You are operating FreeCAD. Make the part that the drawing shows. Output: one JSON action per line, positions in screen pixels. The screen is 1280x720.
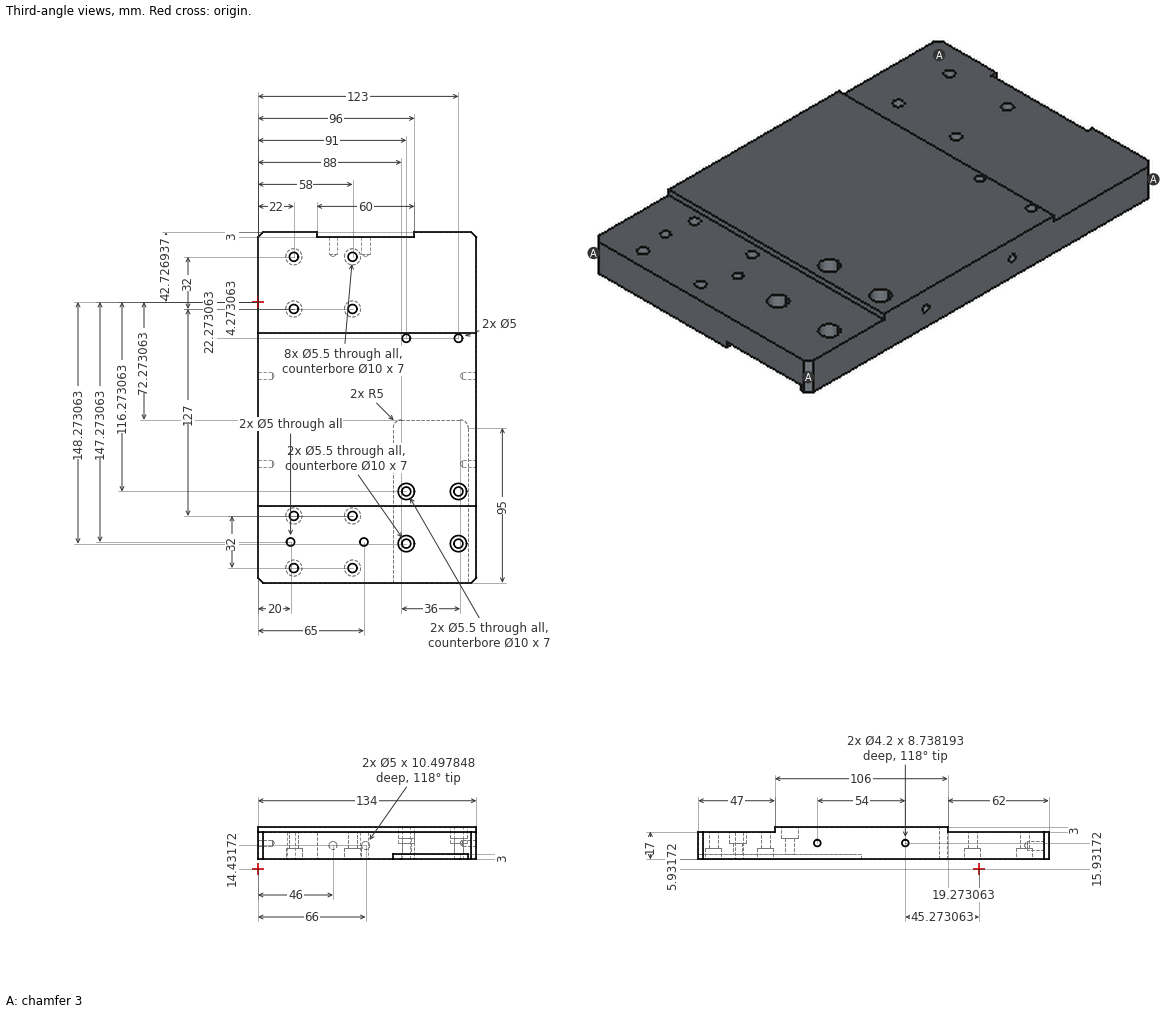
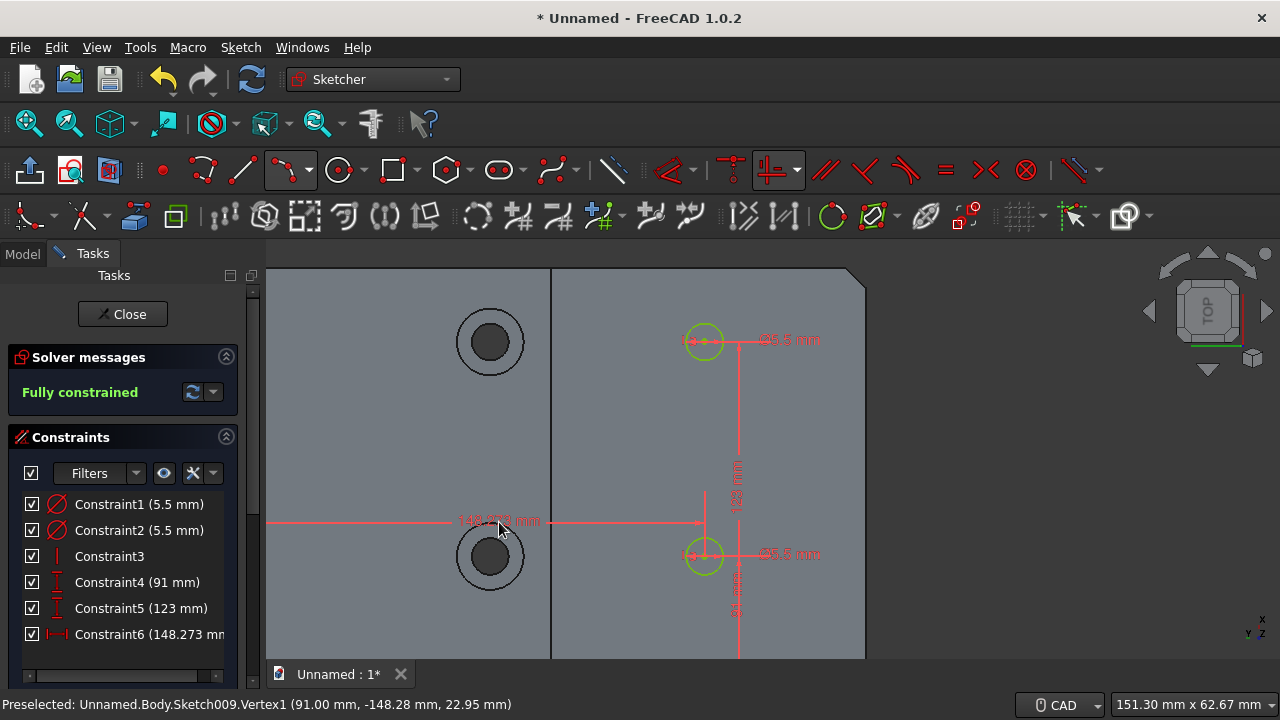
{"action": "left_click", "coordinate": [123, 314]}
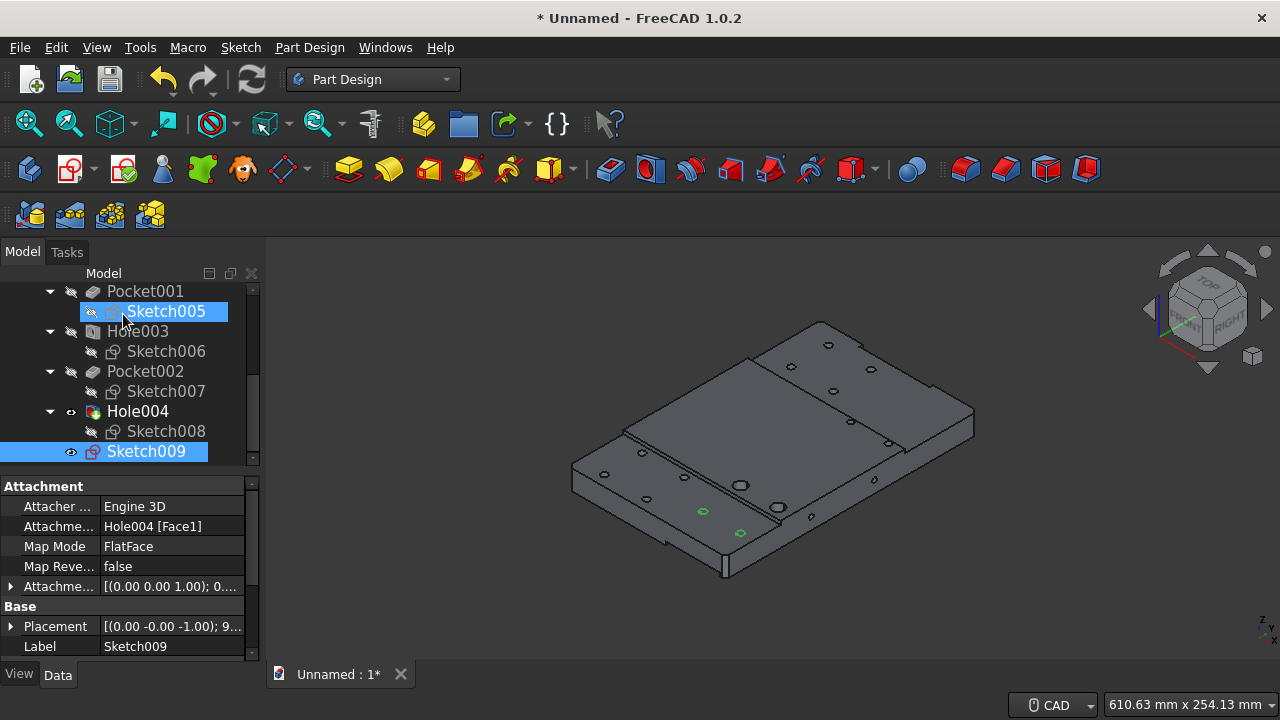
{"action": "left_click", "coordinate": [652, 170]}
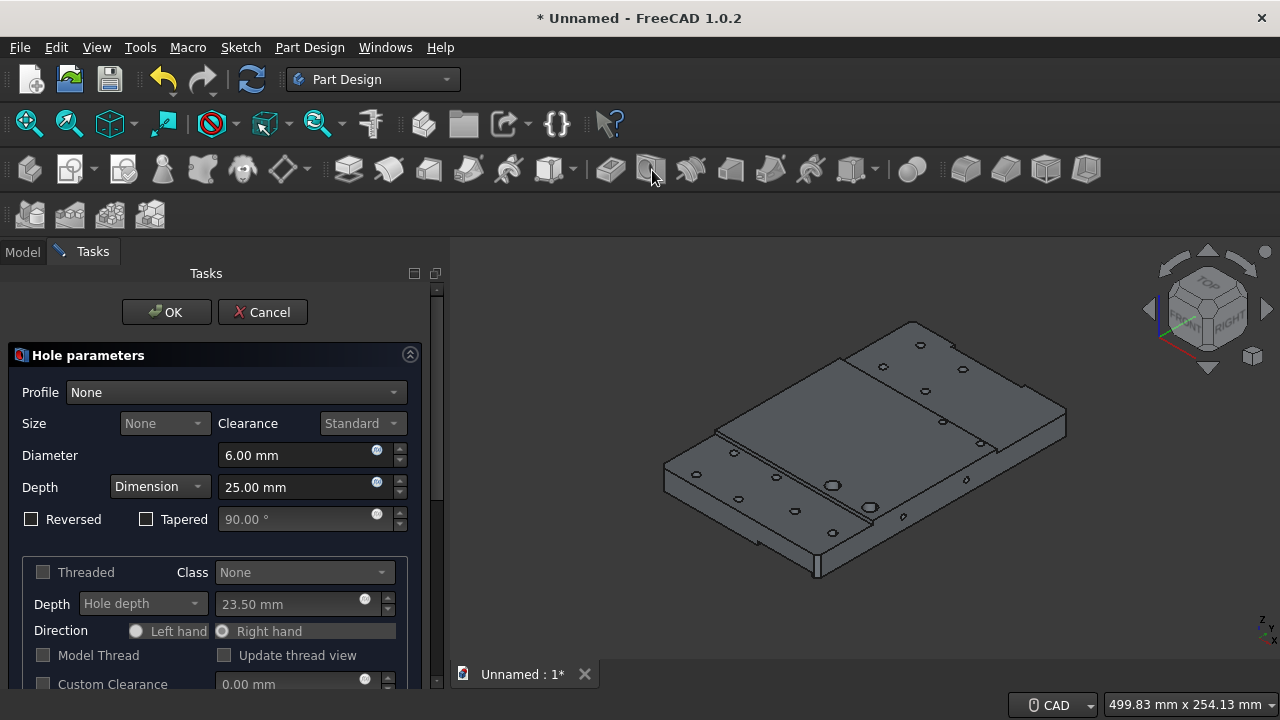
{"action": "triple_click", "coordinate": [305, 455]}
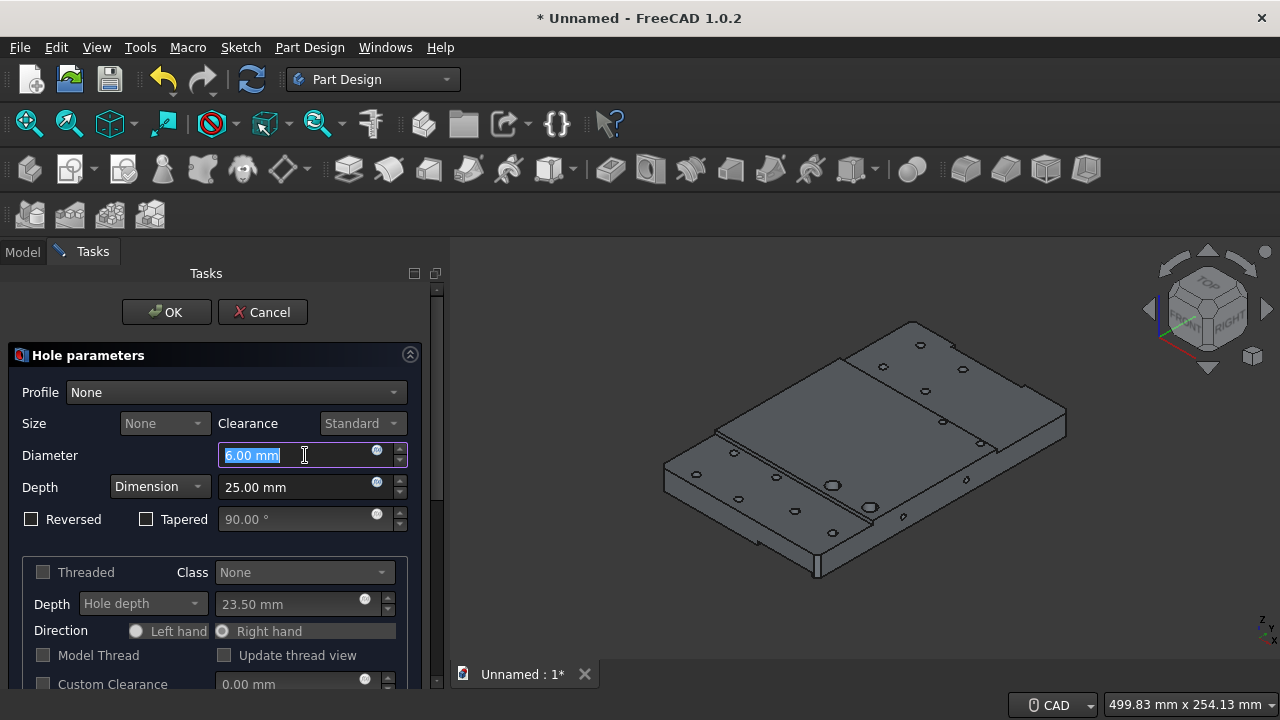
{"action": "type", "text": "5.5"}
{"action": "key", "text": "Tab"}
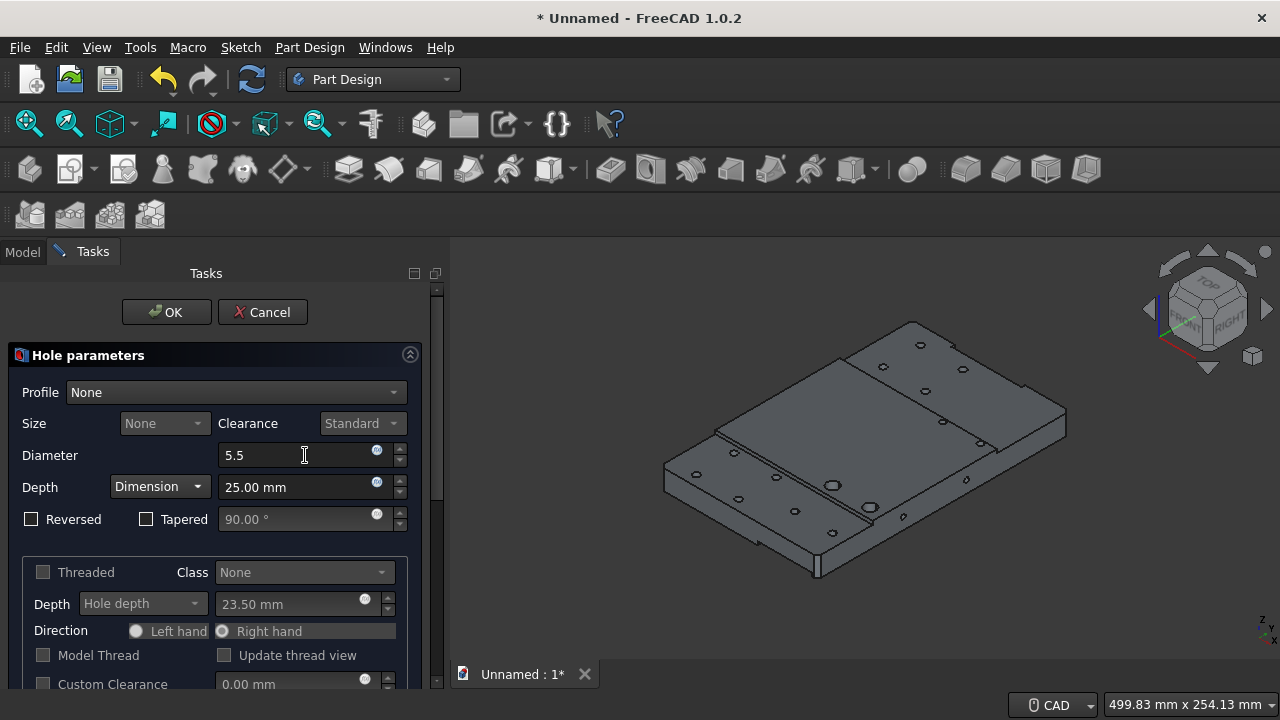
{"action": "left_click", "coordinate": [161, 486]}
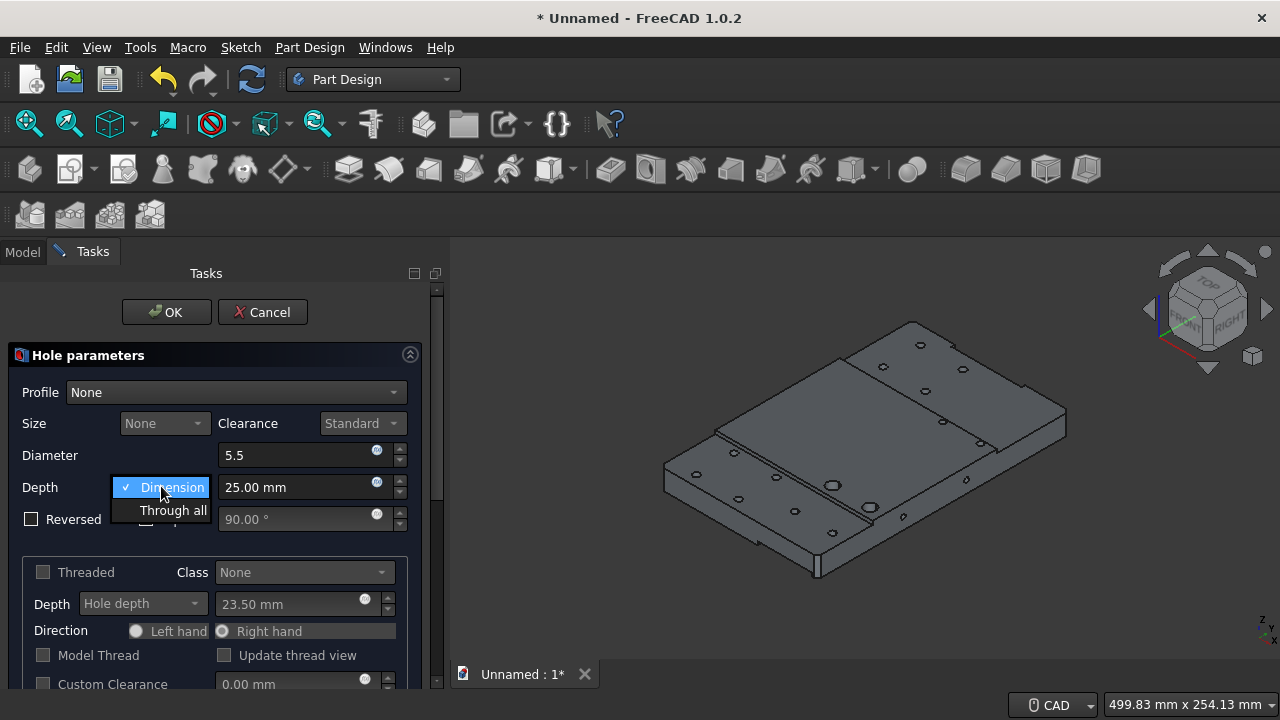
{"action": "left_click", "coordinate": [160, 510]}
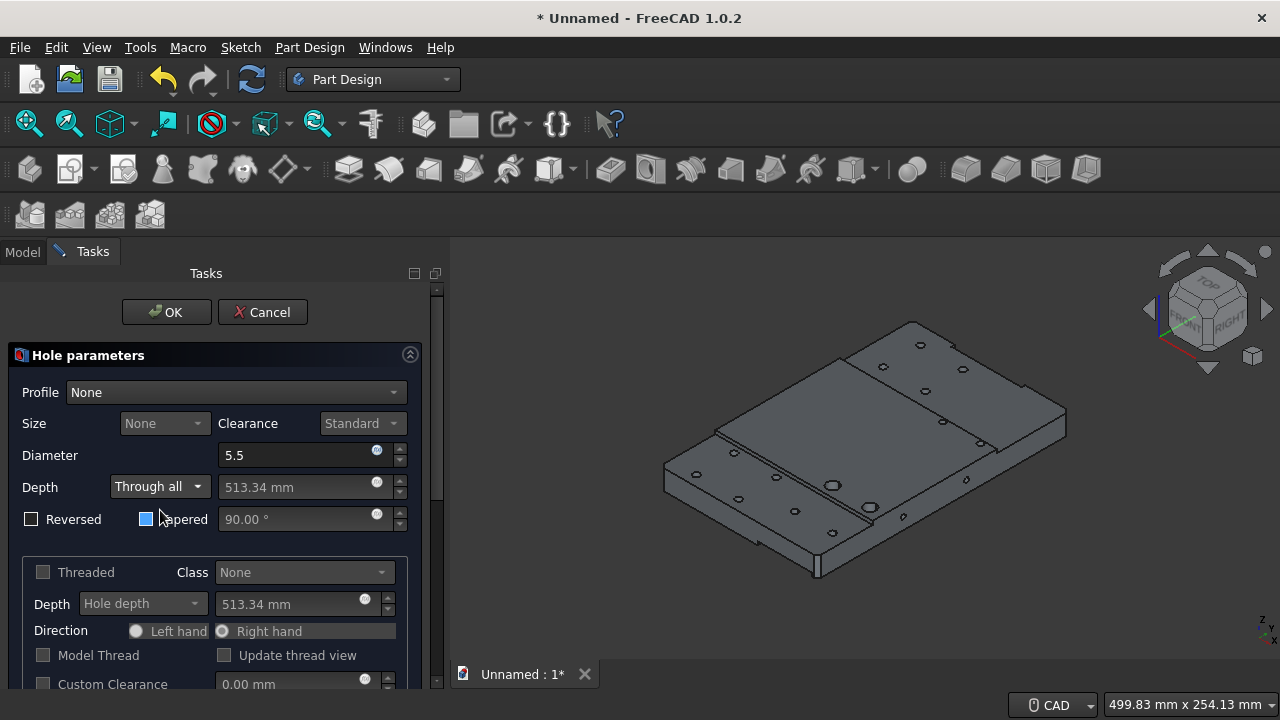
{"action": "scroll", "coordinate": [437, 486], "scroll_direction": "down", "scroll_amount": 3}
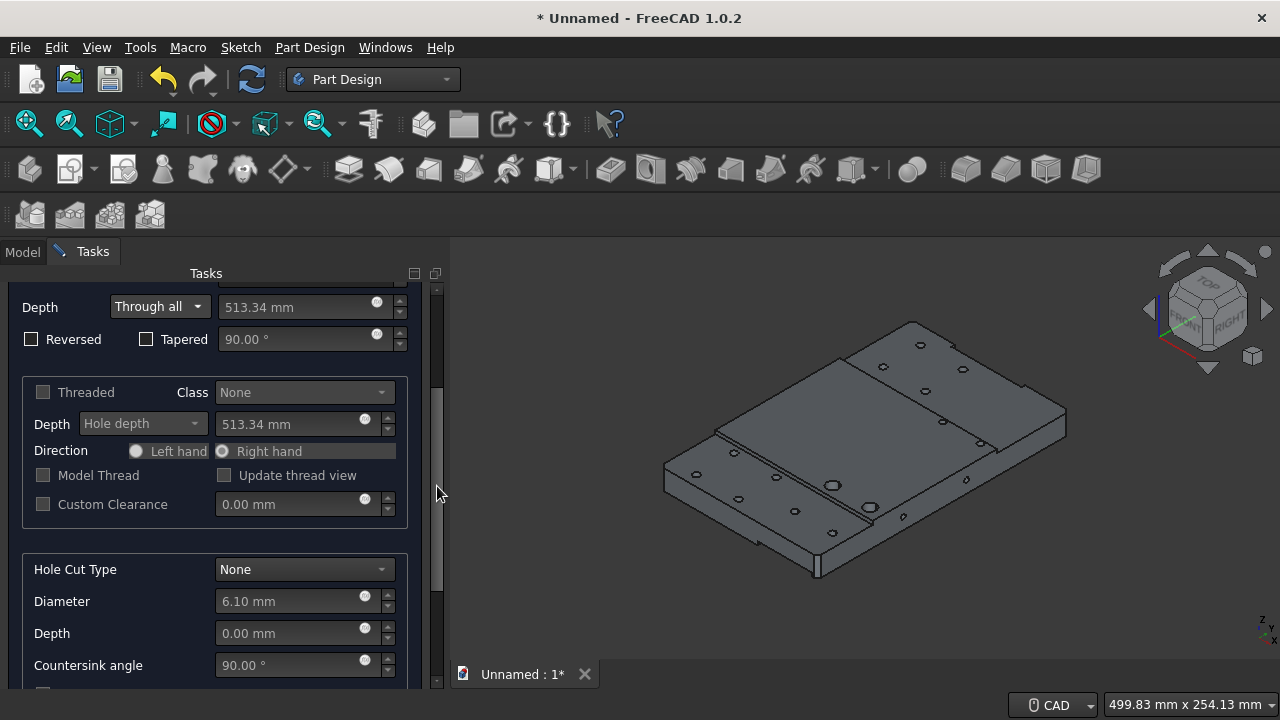
{"action": "left_click", "coordinate": [306, 570]}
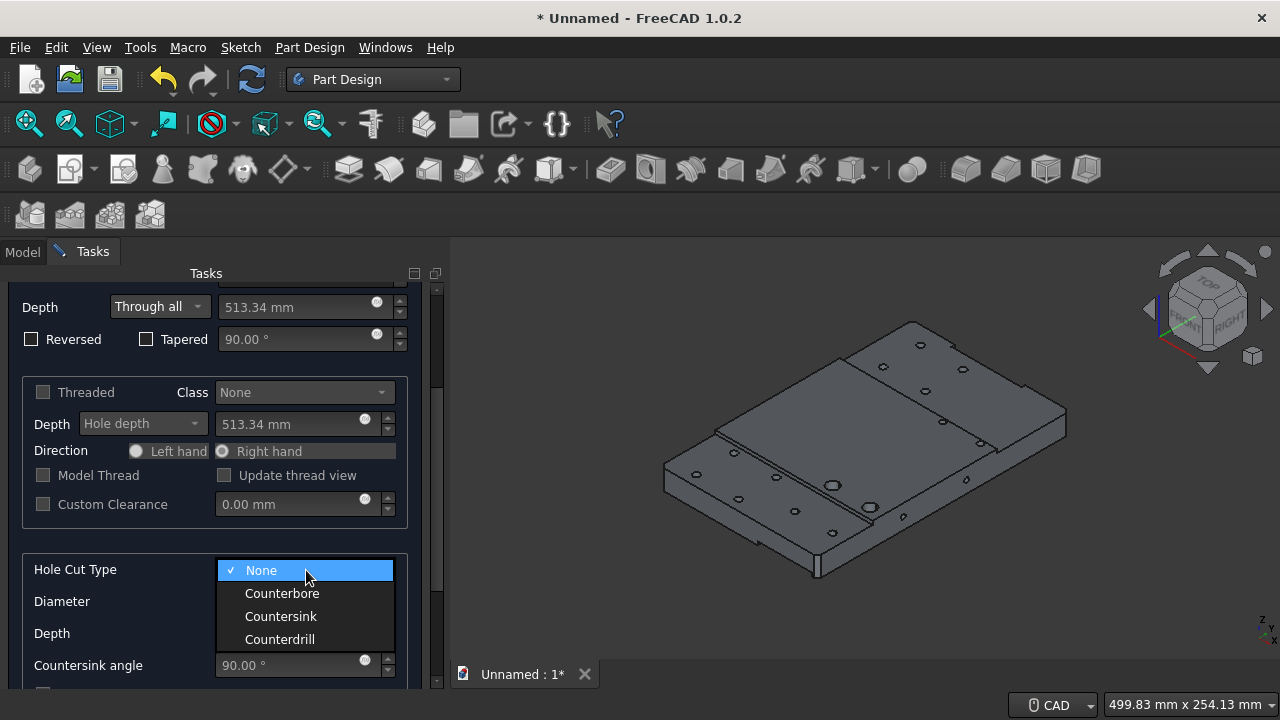
{"action": "left_click", "coordinate": [304, 594]}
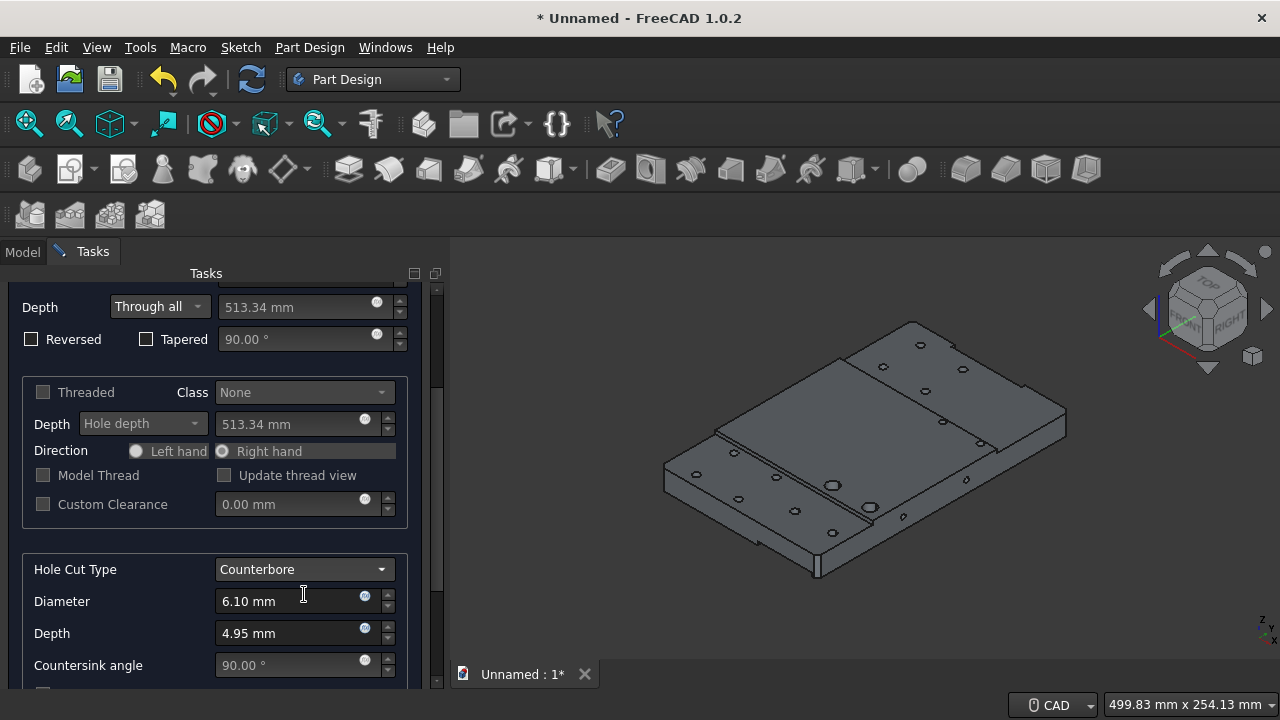
{"action": "triple_click", "coordinate": [298, 601]}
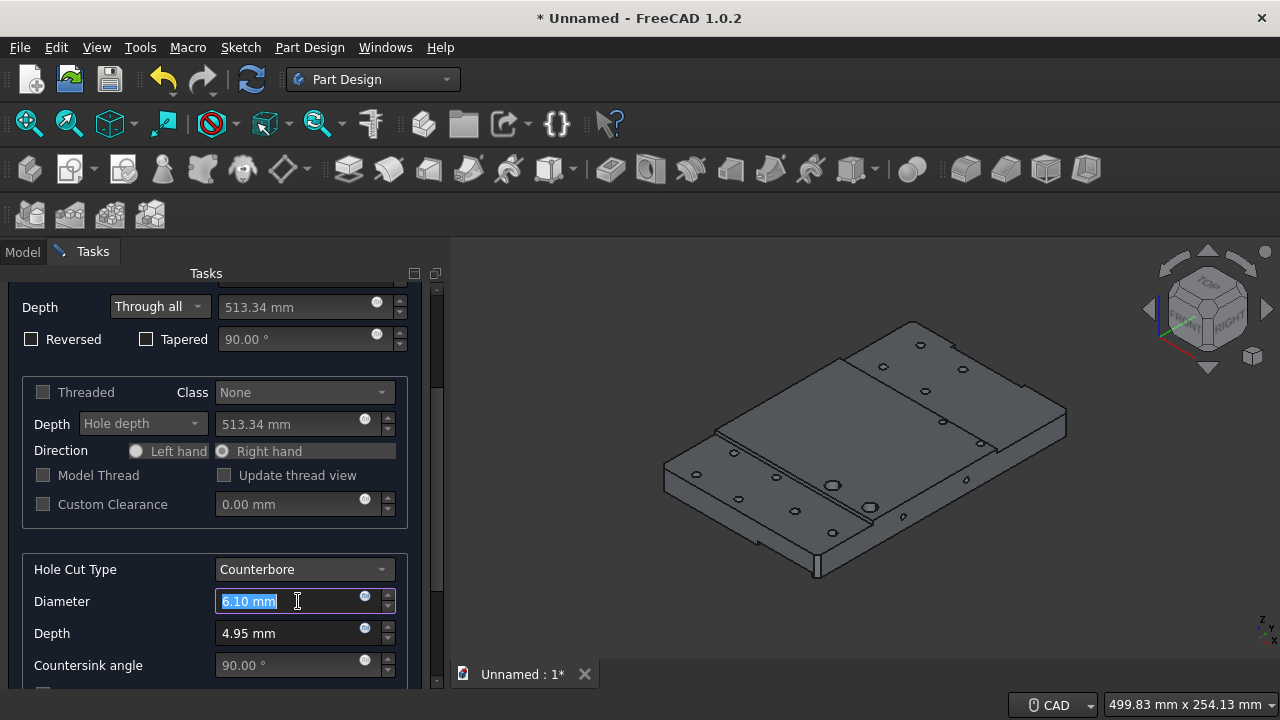
{"action": "type", "text": "10"}
{"action": "key", "text": "Tab"}